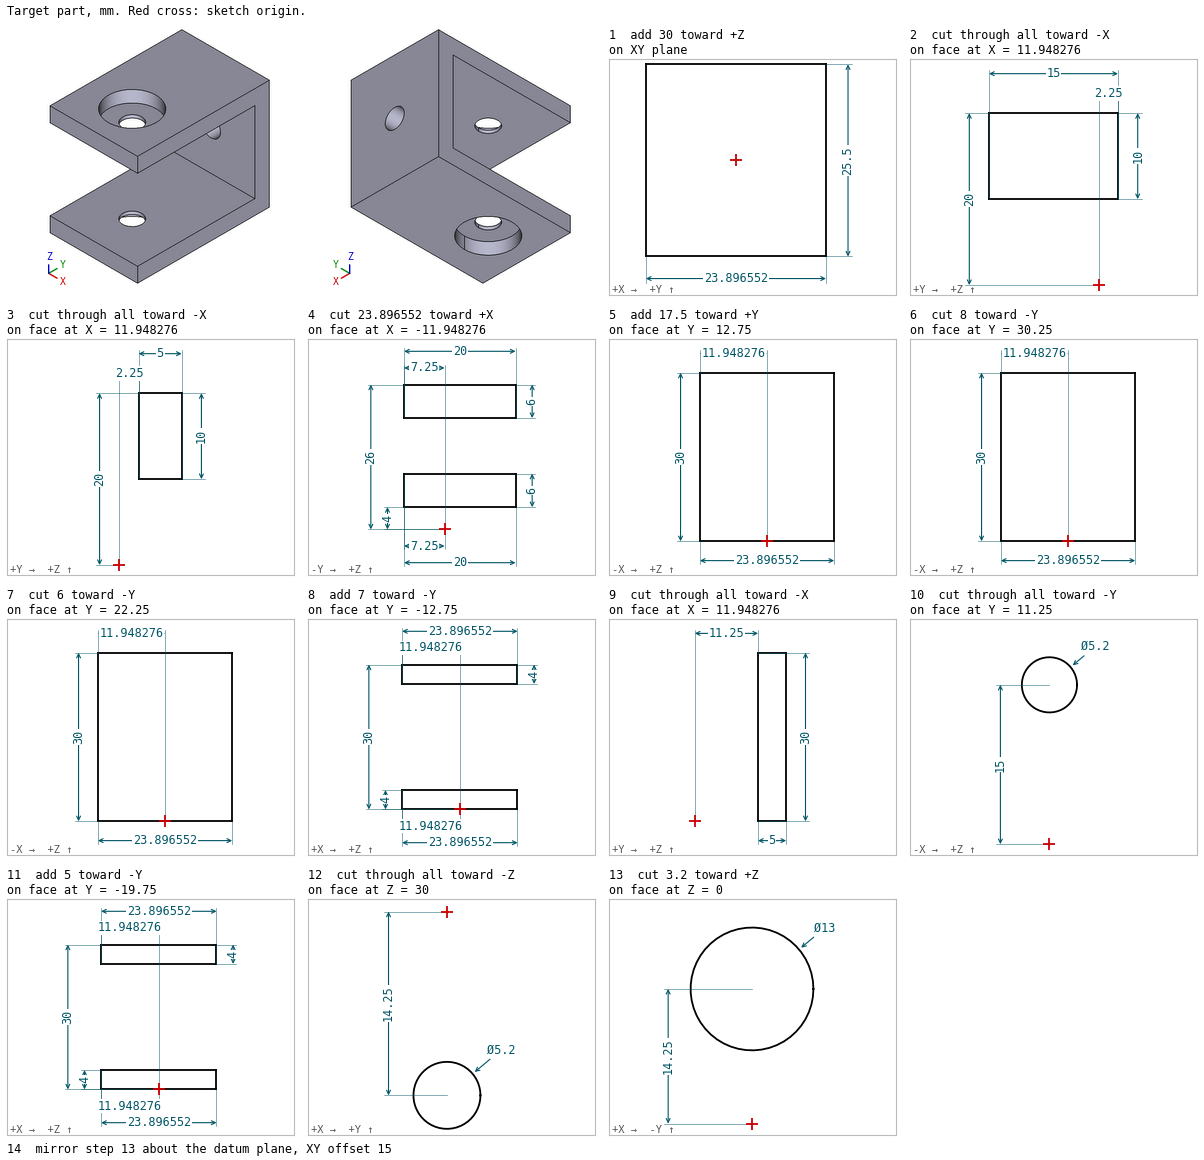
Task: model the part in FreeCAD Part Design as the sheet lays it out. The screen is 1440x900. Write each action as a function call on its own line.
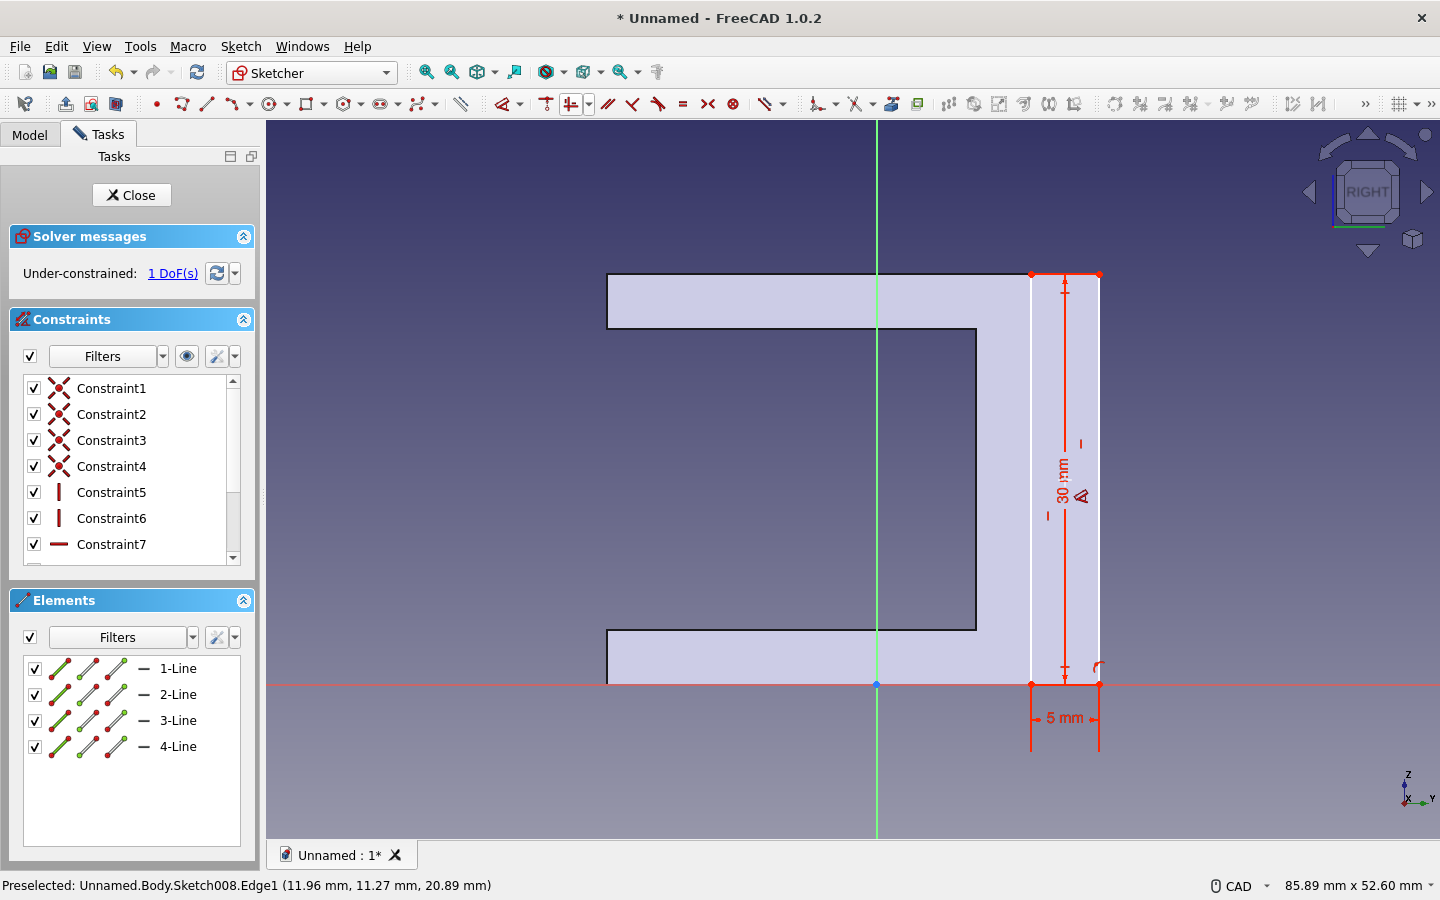
click(1031, 274)
click(954, 719)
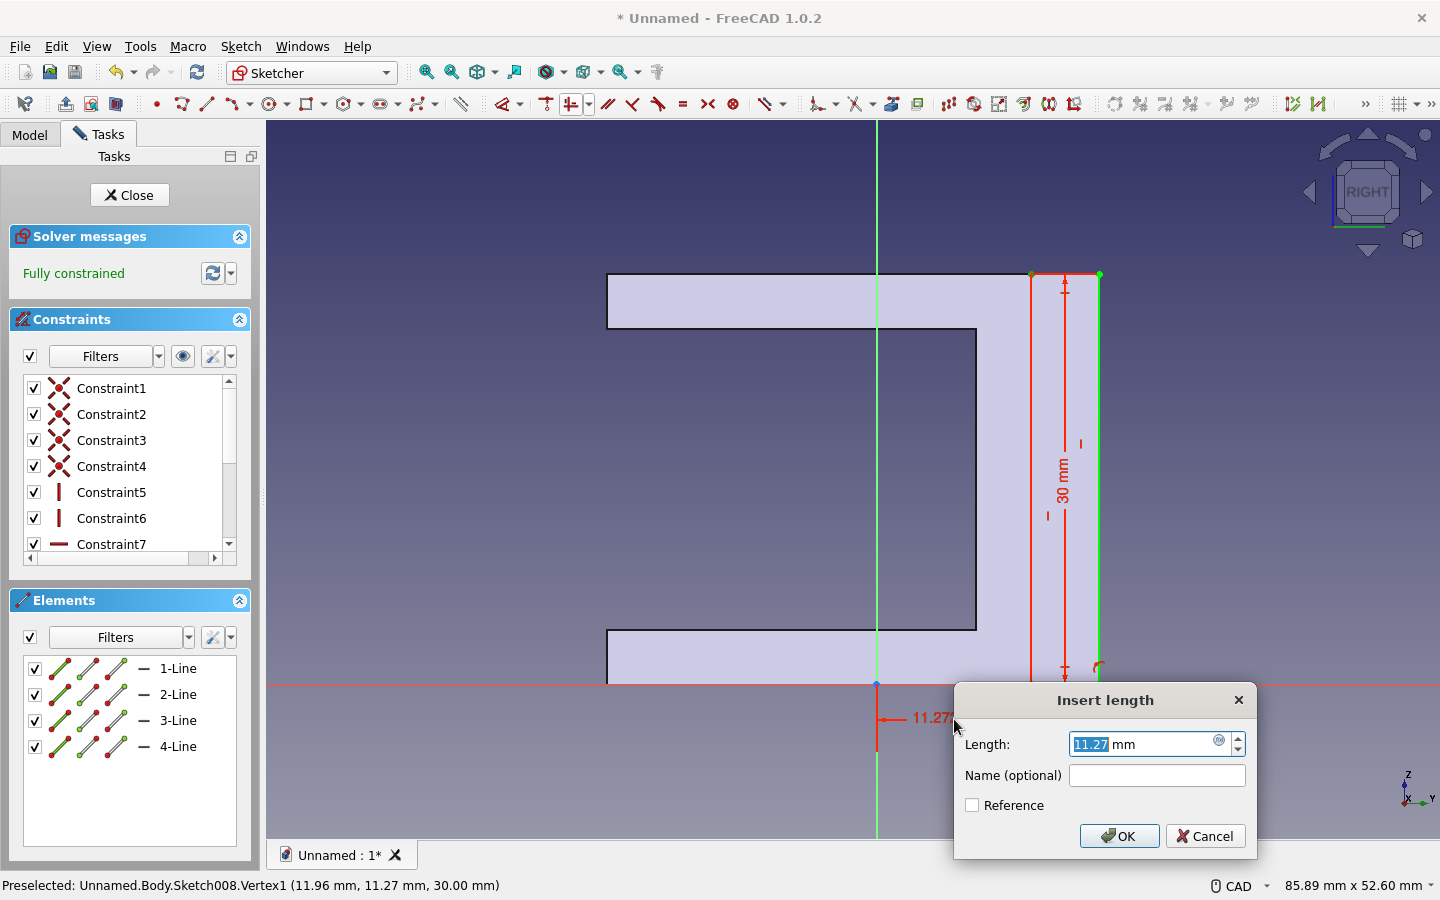
text(11.25)
key(Return)
key(Escape)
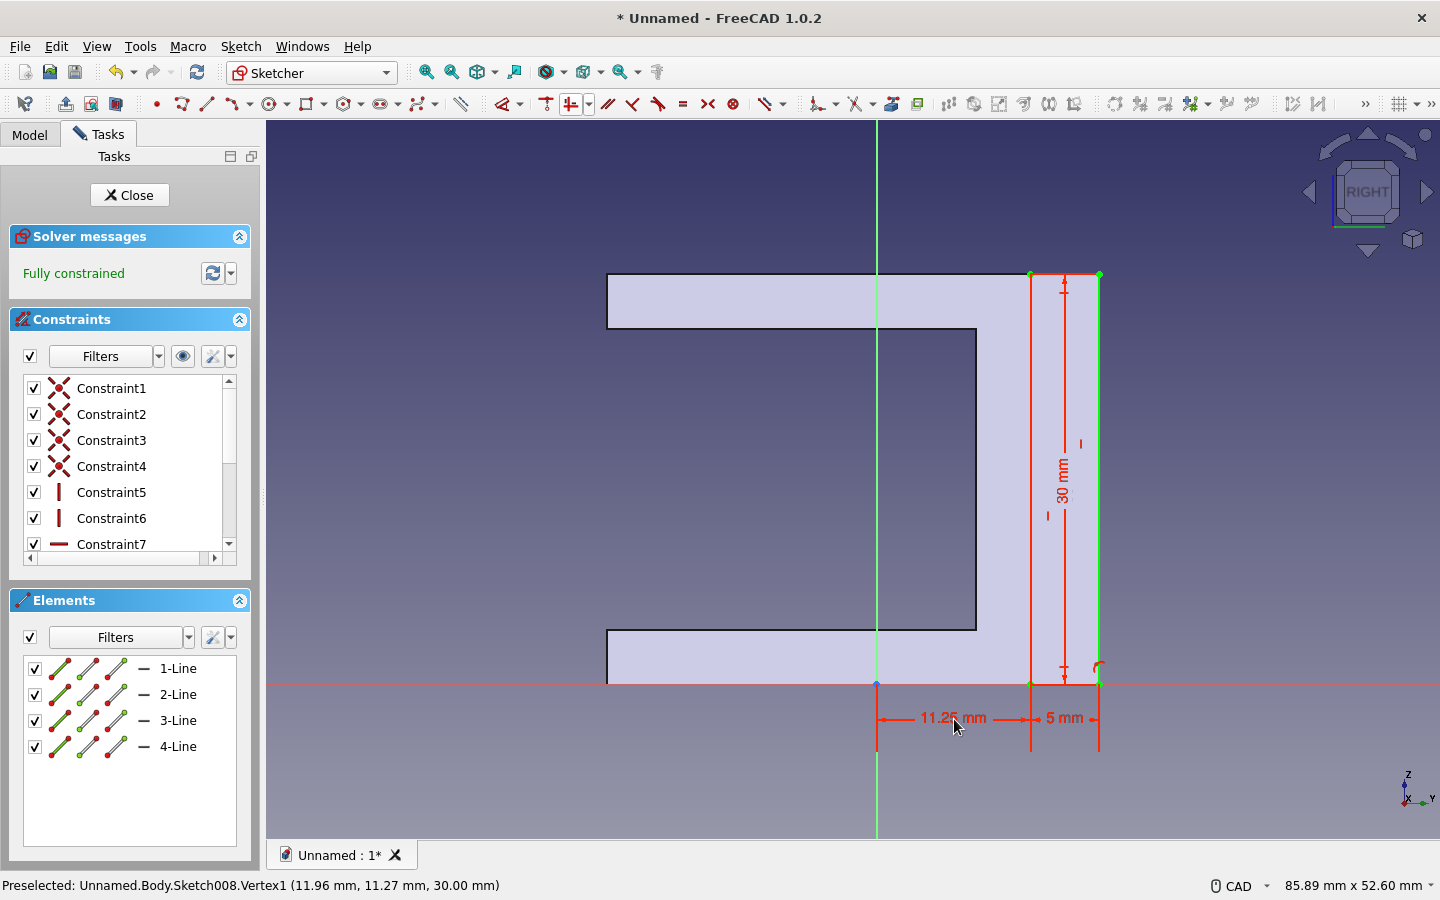
click(130, 195)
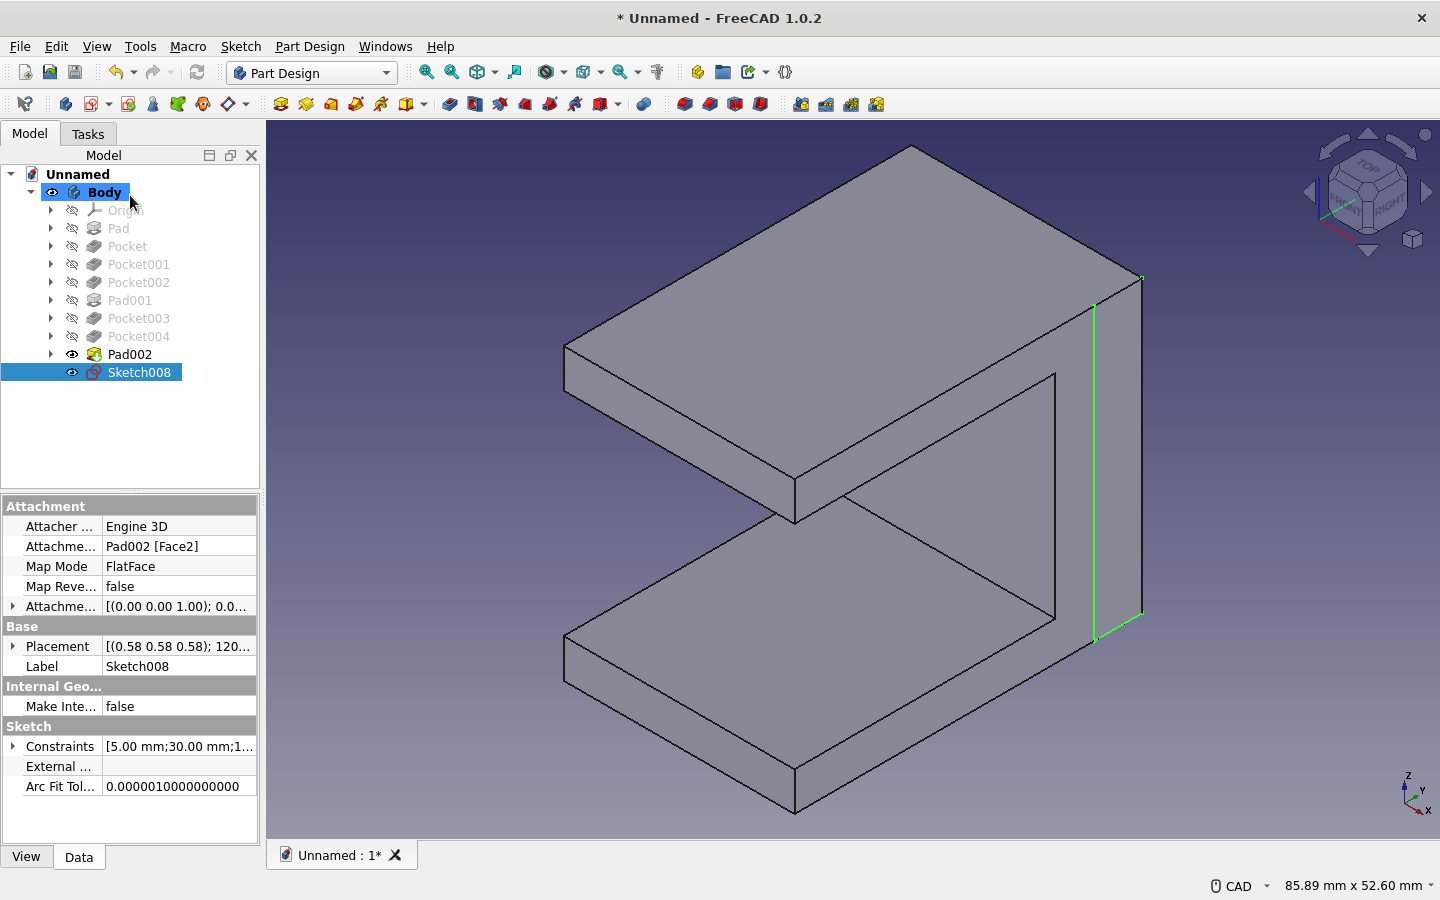
click(450, 104)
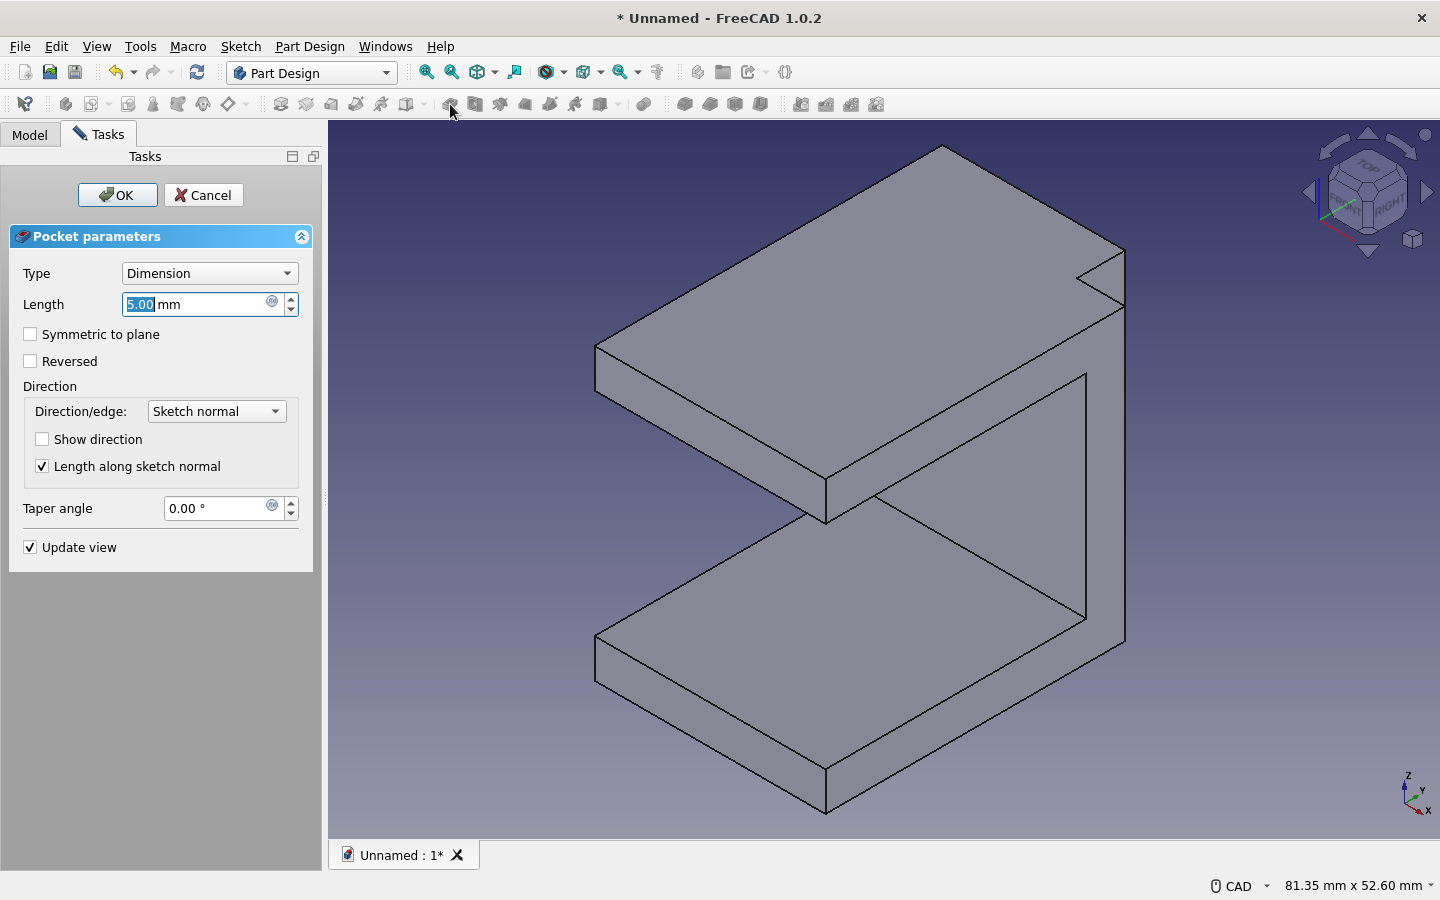
click(210, 274)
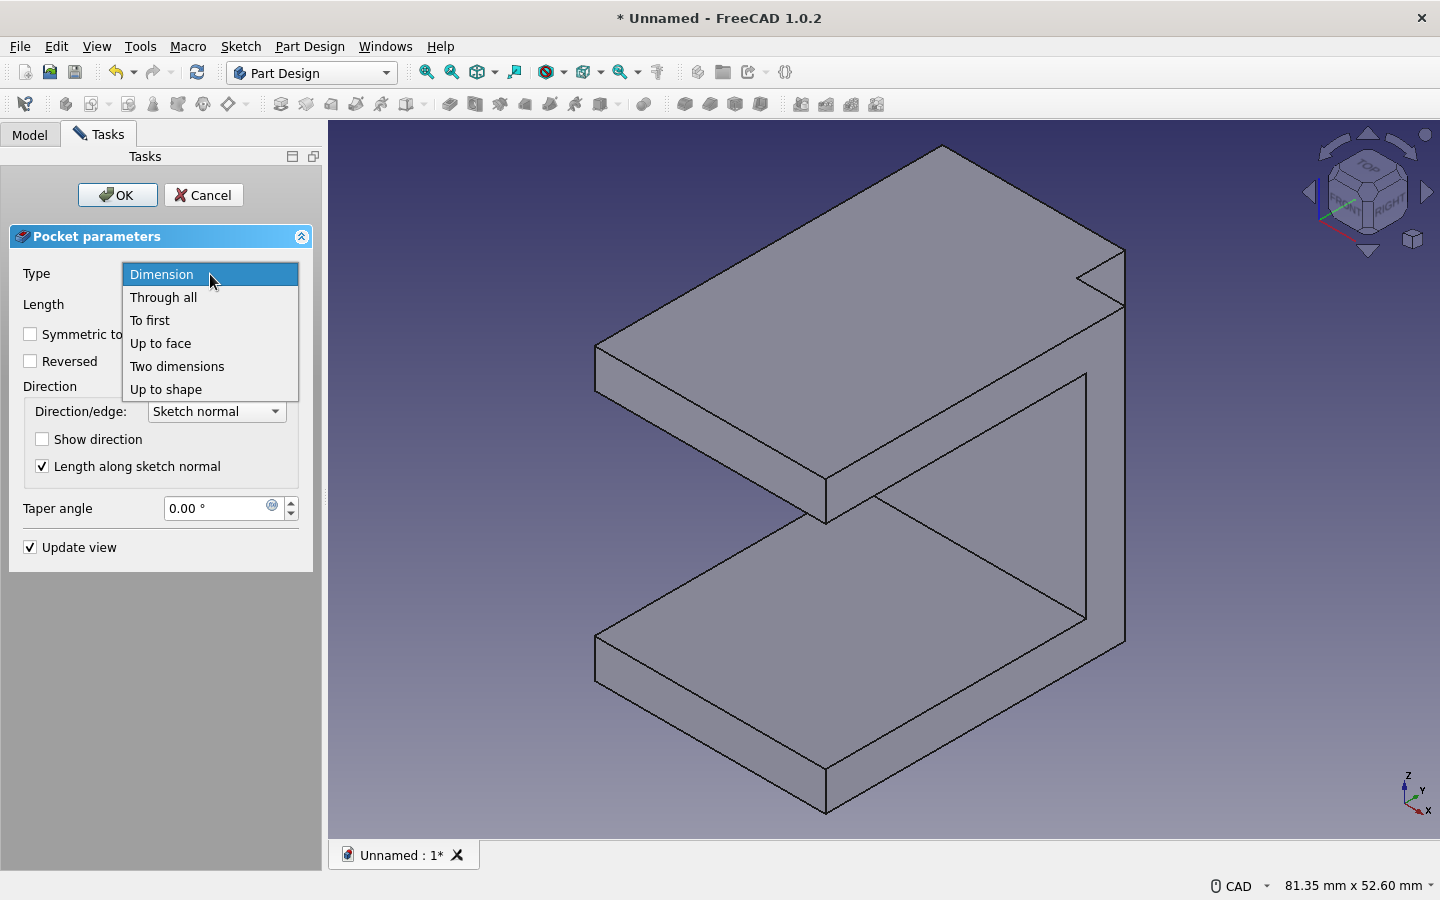
click(208, 298)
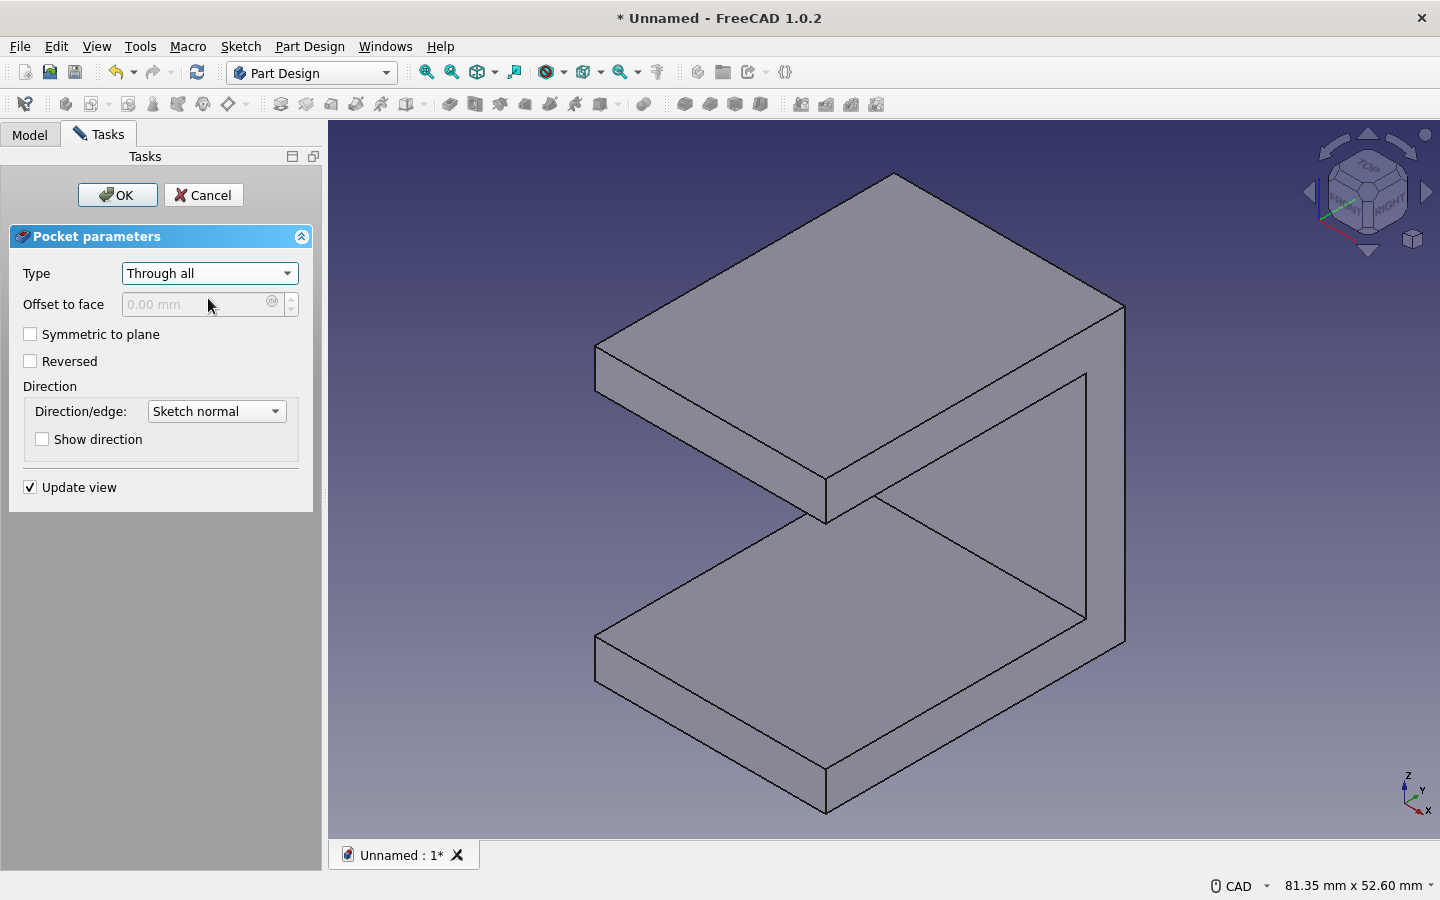
click(118, 195)